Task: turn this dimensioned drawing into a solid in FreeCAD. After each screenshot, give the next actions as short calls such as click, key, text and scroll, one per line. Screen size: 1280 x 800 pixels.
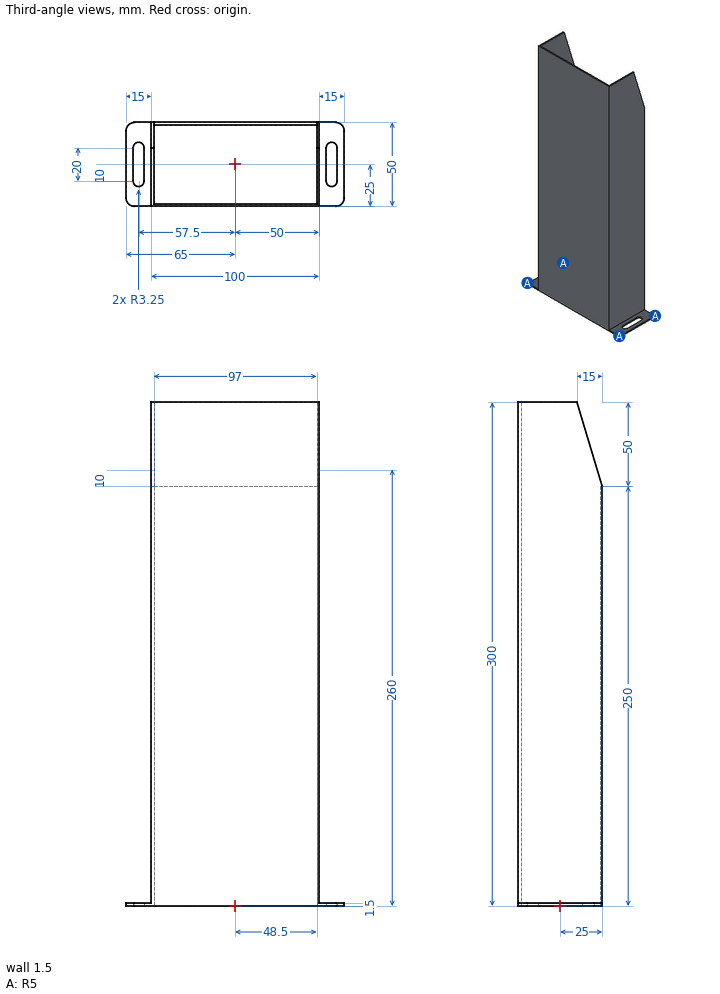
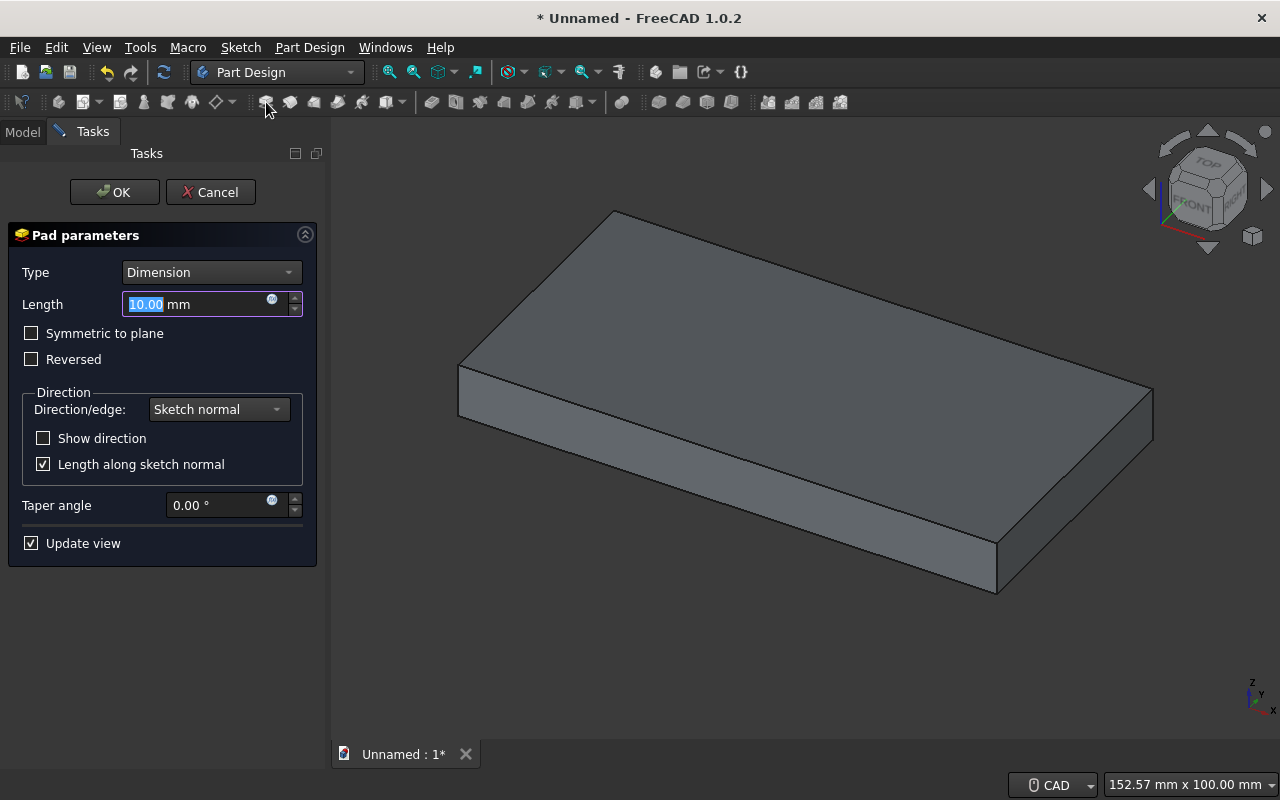
text(300)
key(Tab)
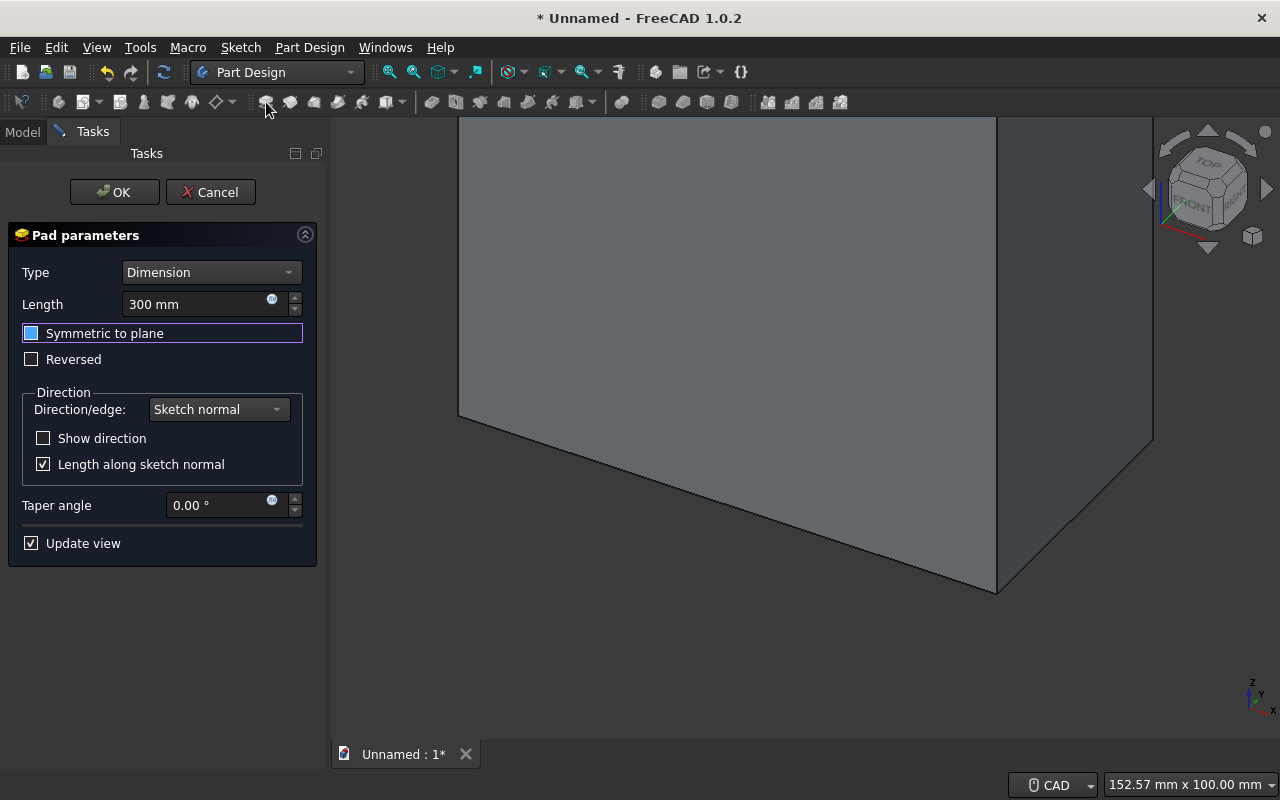
click(115, 192)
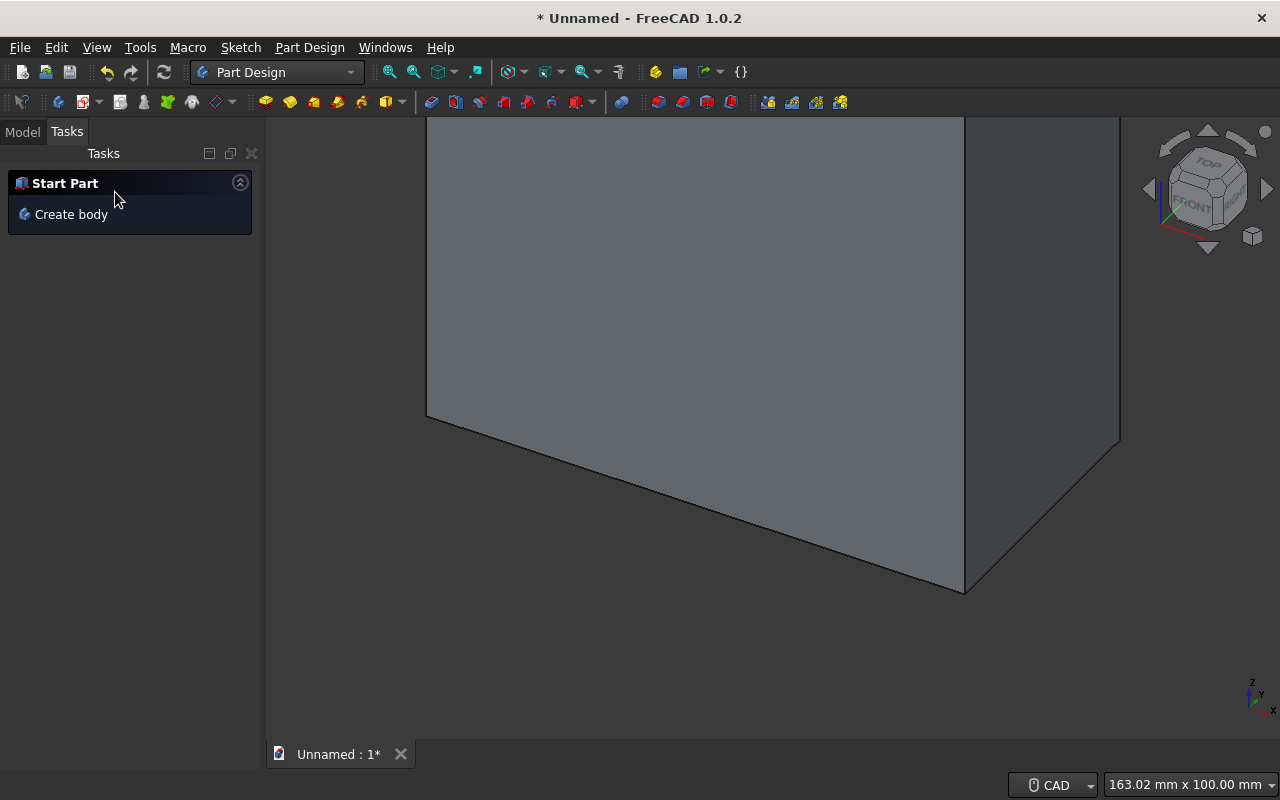
click(390, 72)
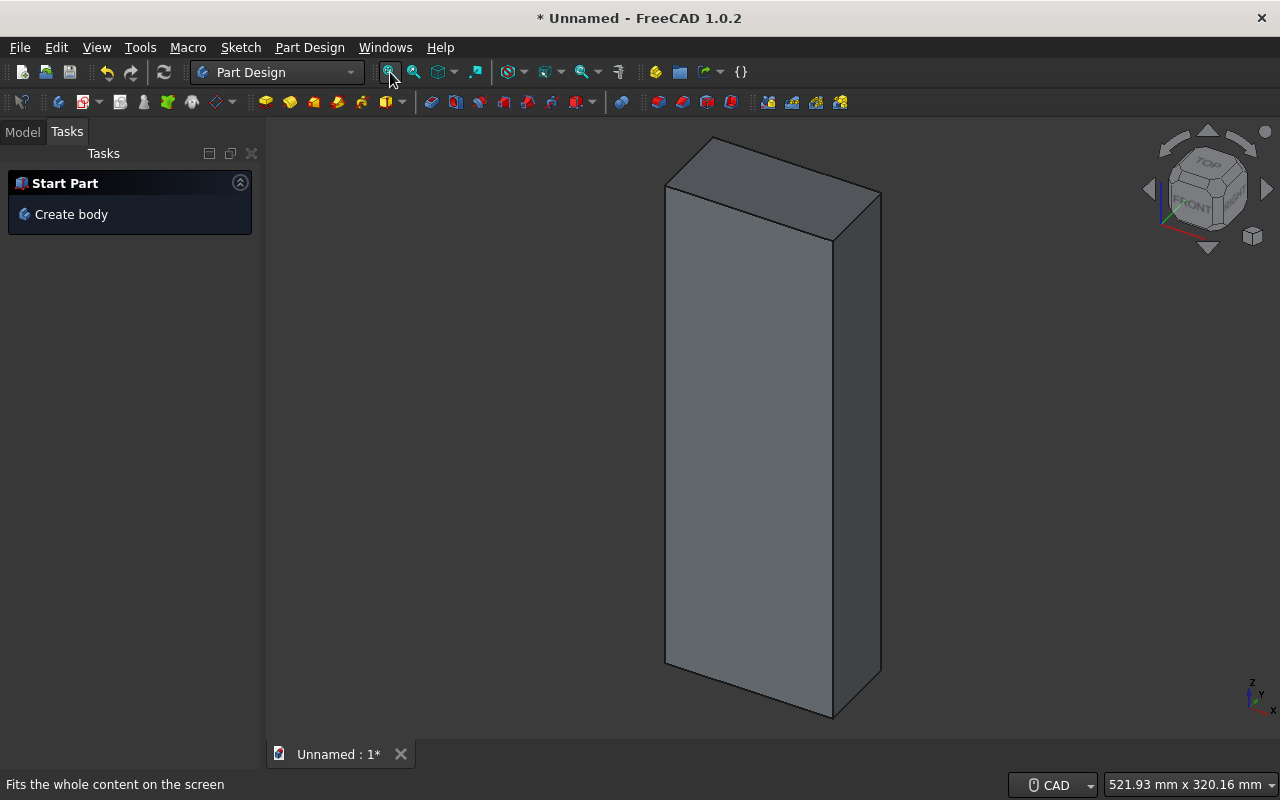
click(797, 196)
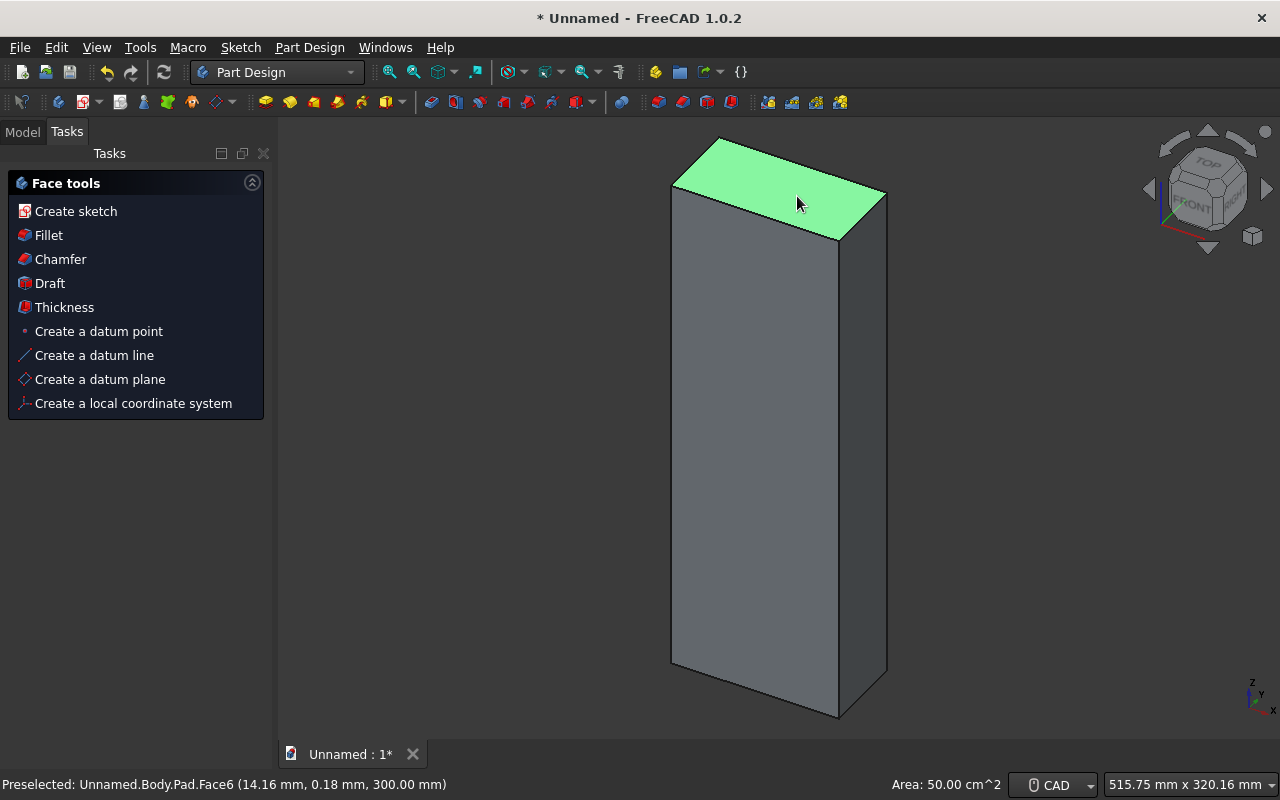
key(0)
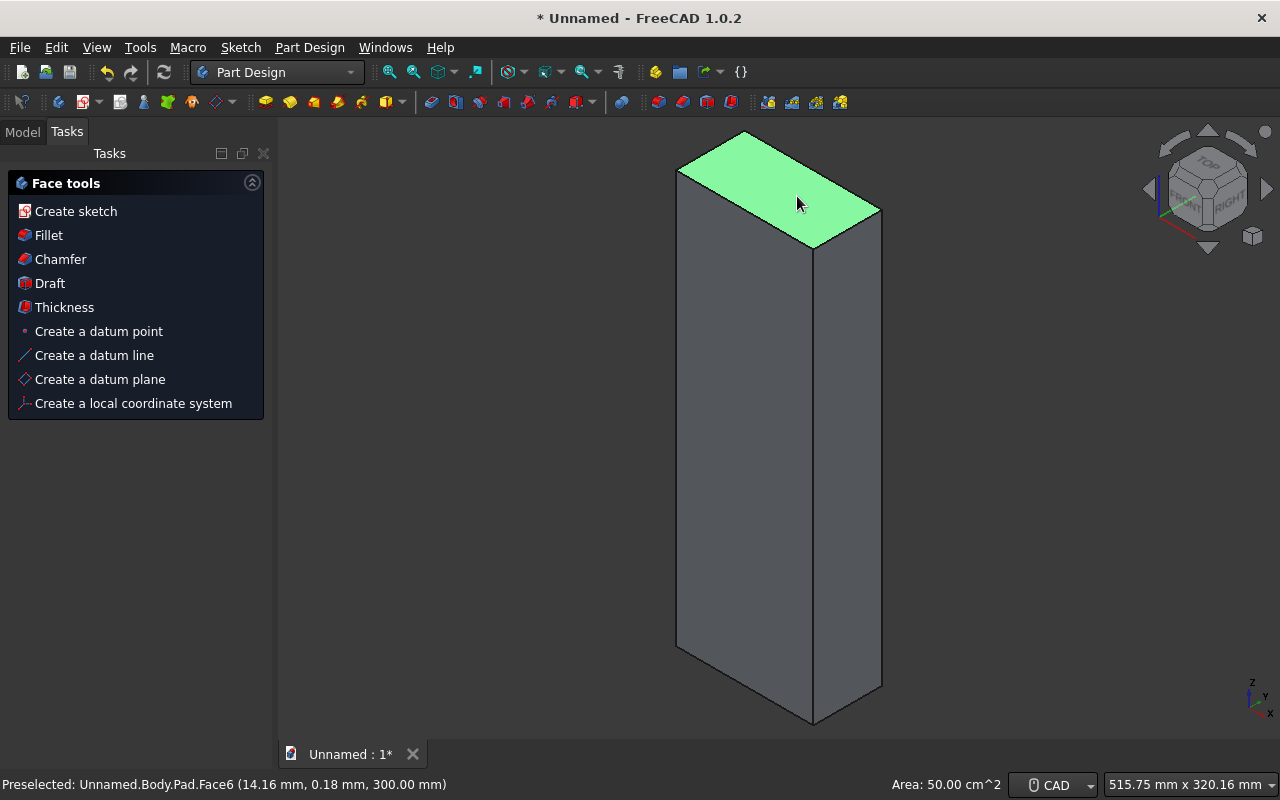
key(2)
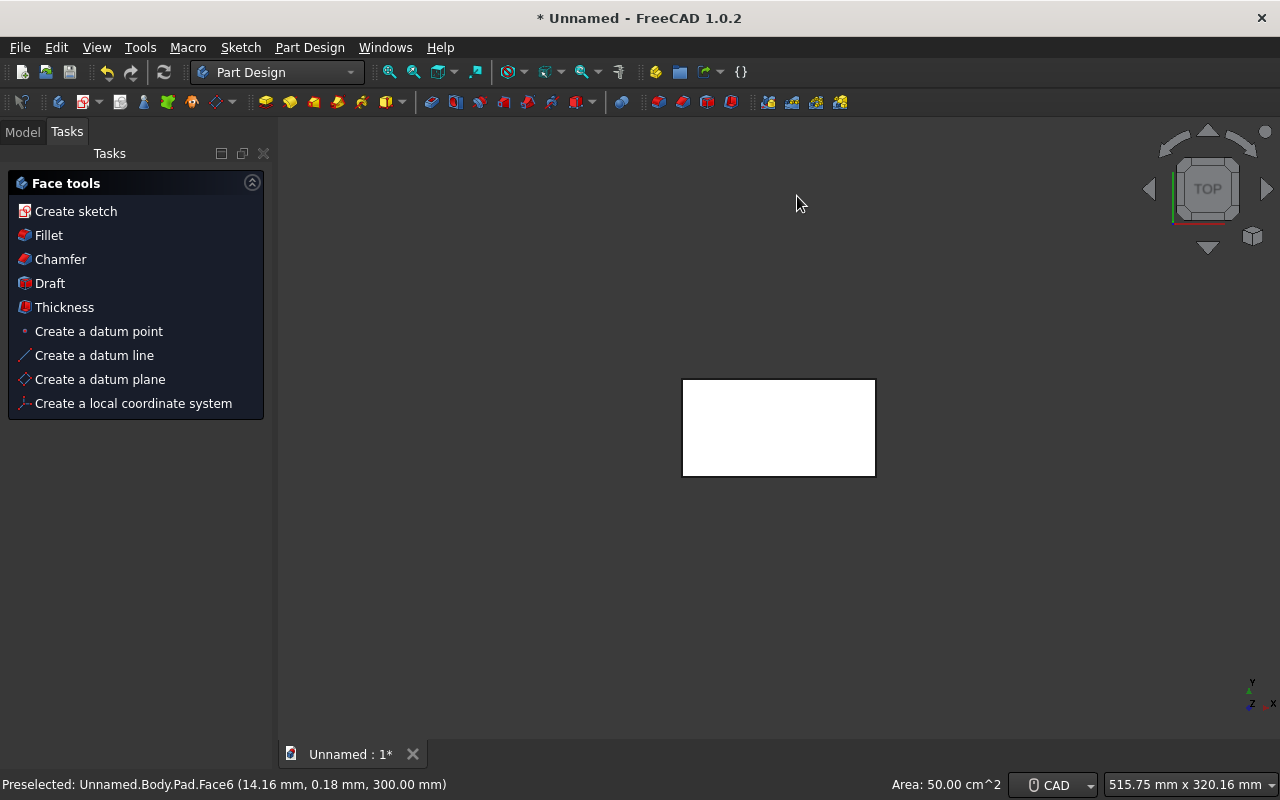
click(390, 72)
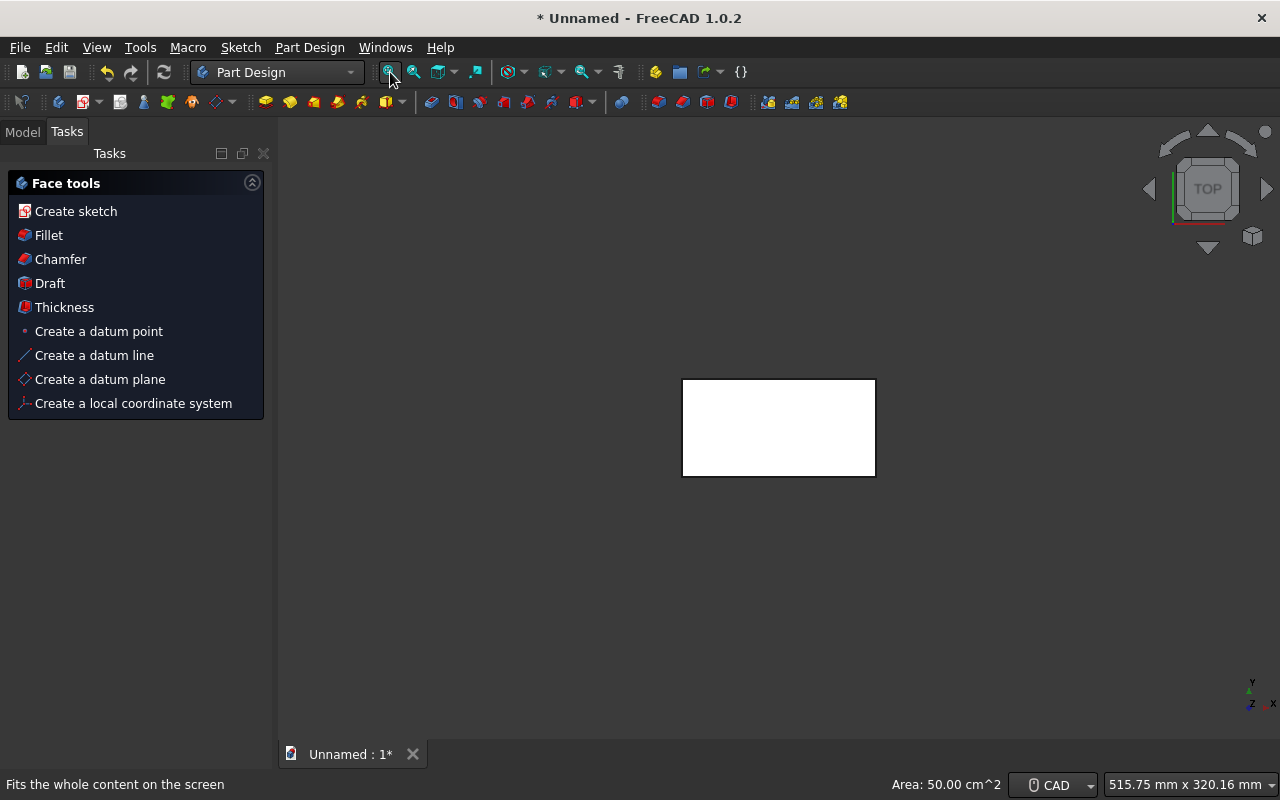
key(1)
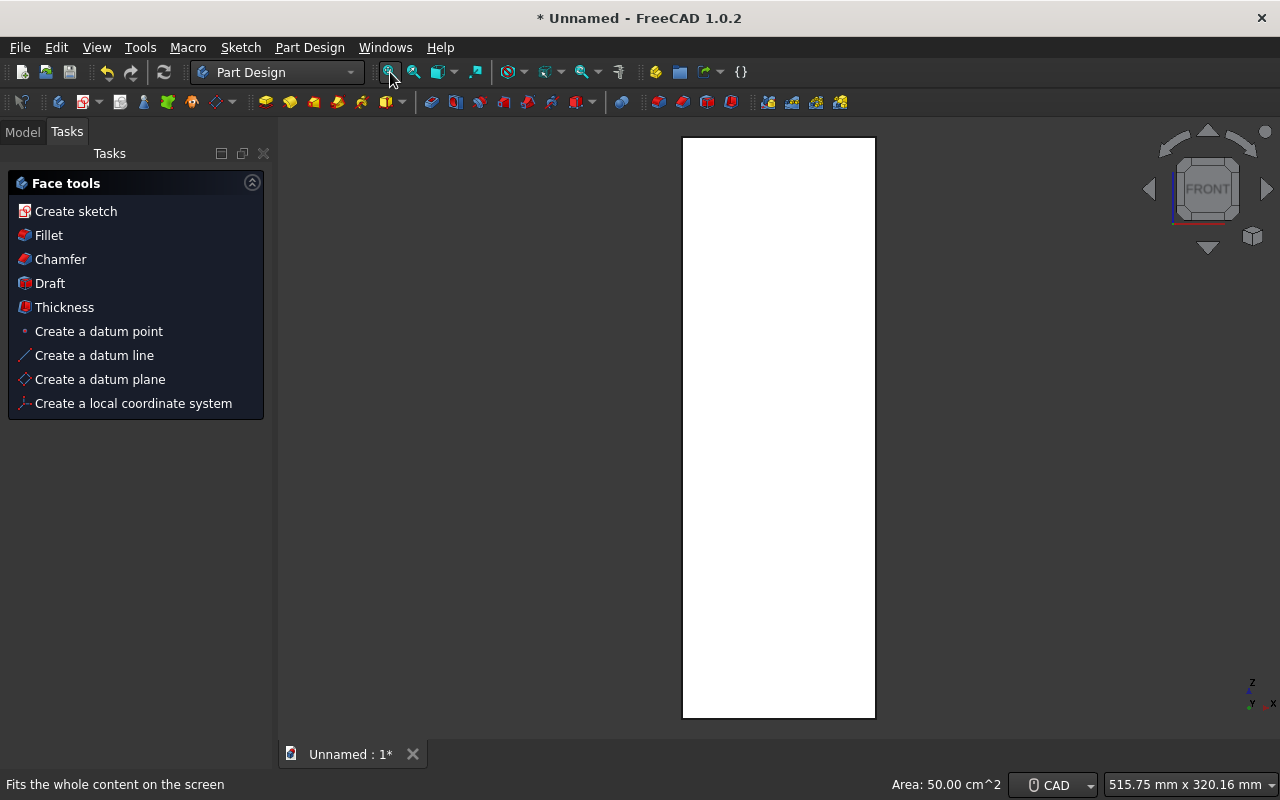
key(3)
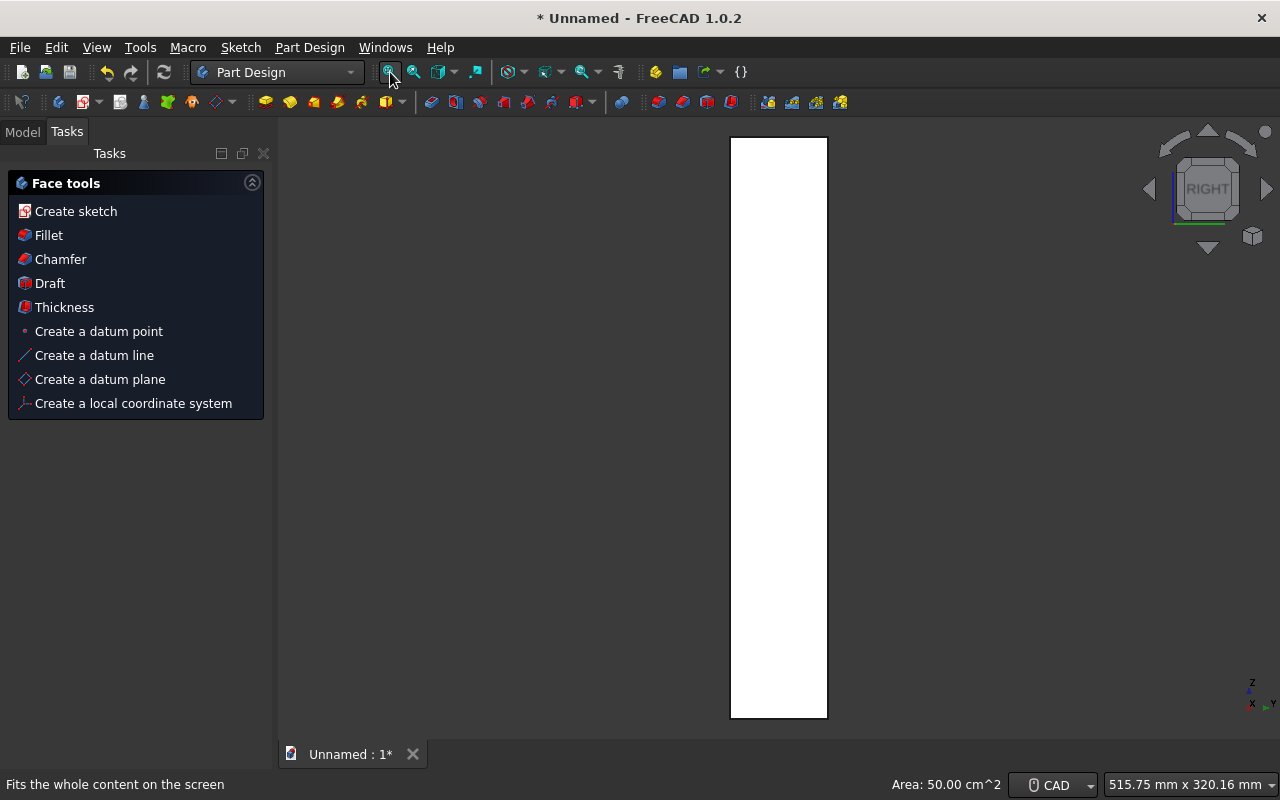
key(5)